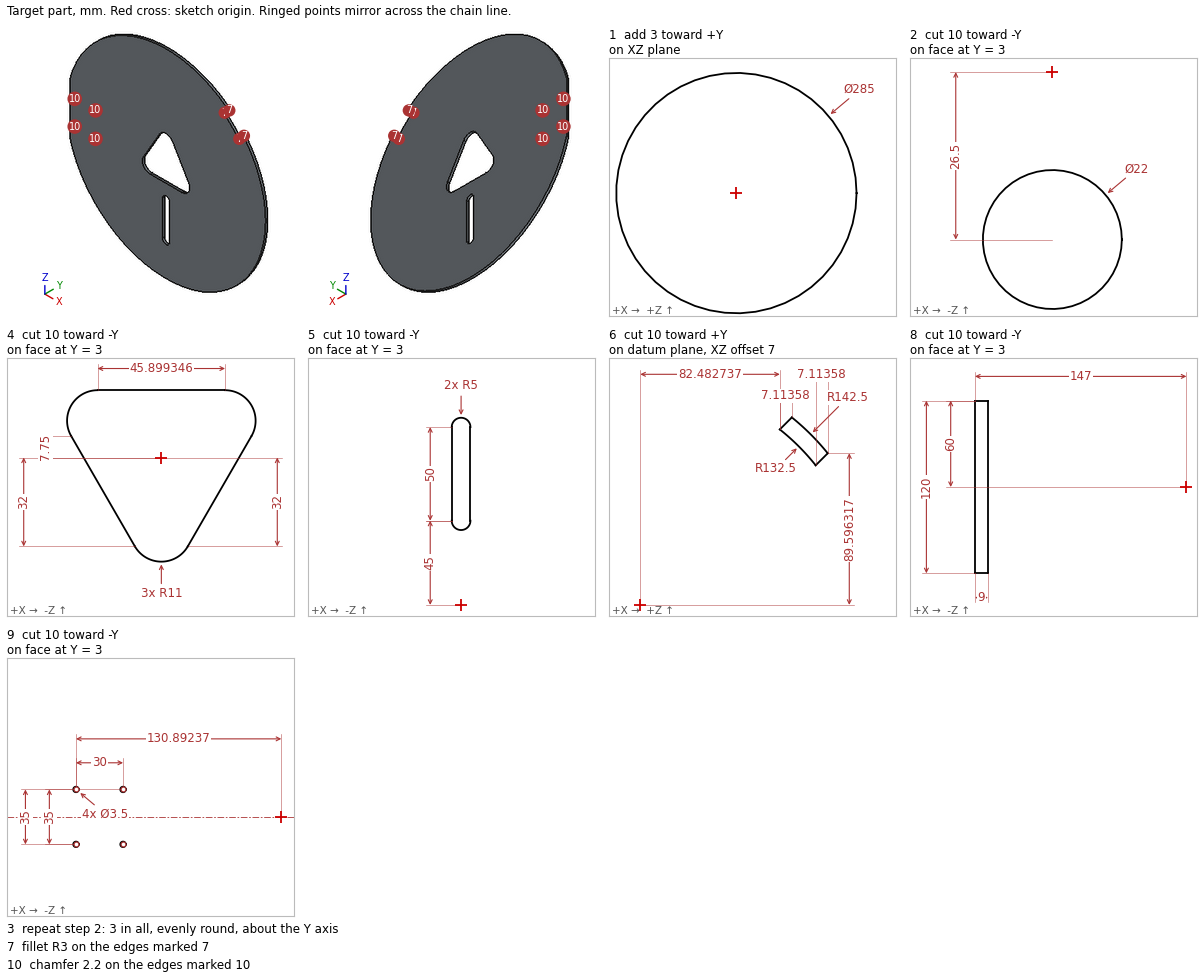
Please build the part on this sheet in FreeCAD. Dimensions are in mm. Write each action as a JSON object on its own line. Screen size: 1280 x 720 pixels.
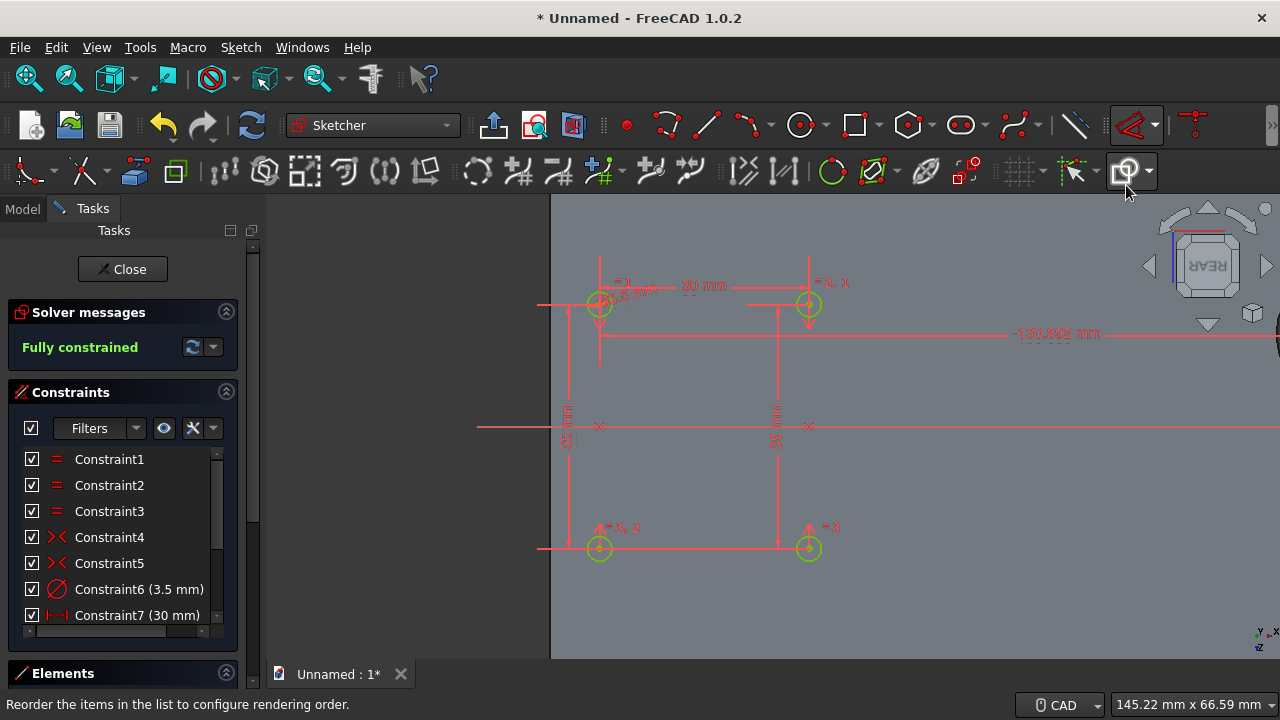
{"action": "left_click", "coordinate": [123, 269]}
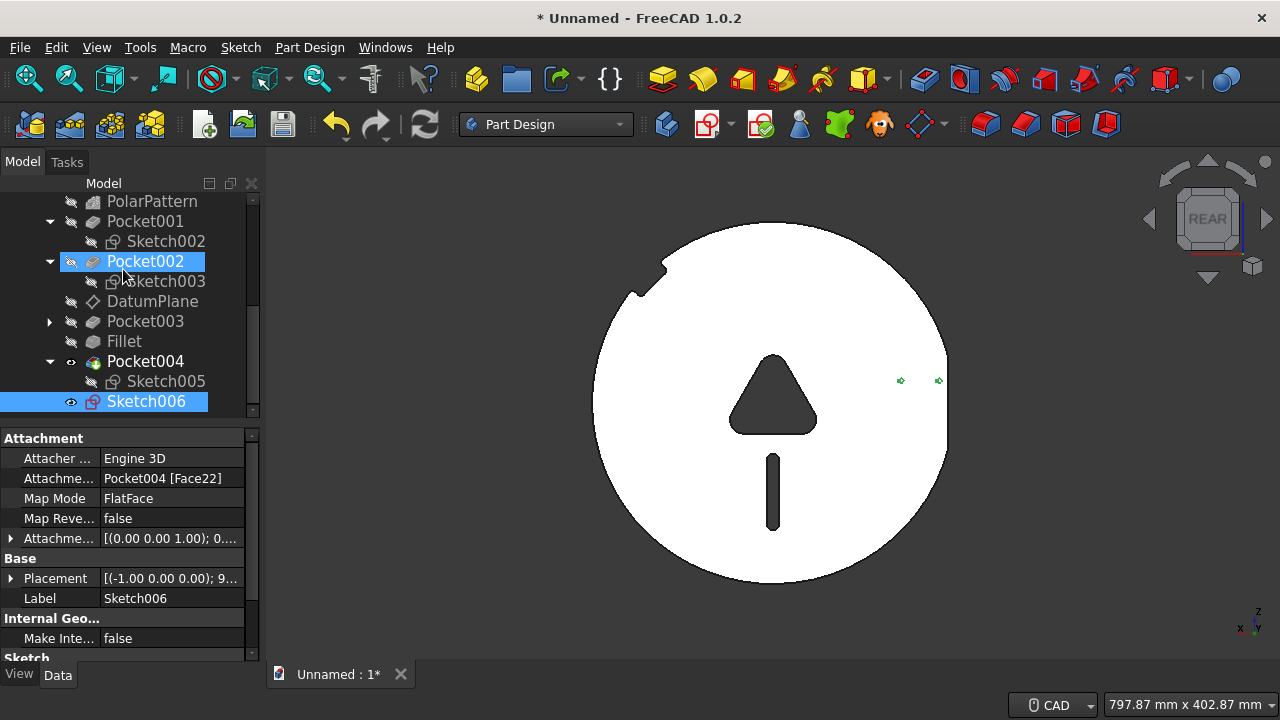
{"action": "left_click", "coordinate": [926, 80]}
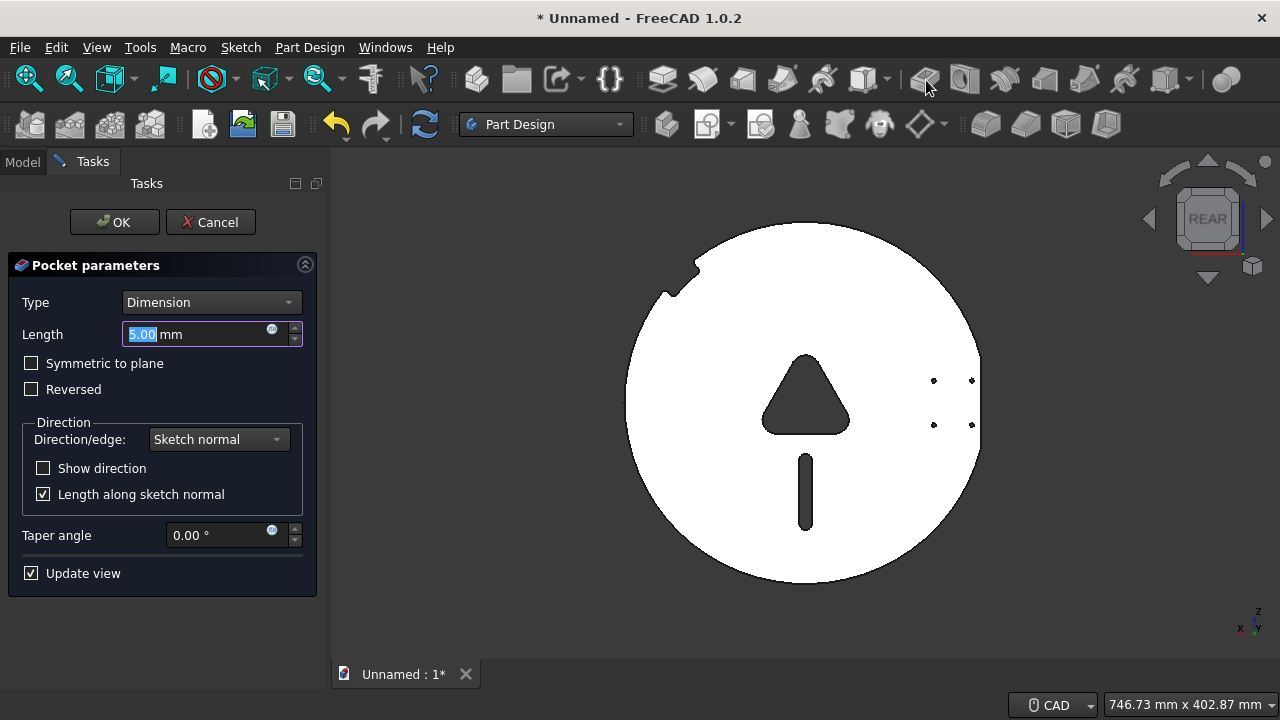
{"action": "type", "text": "10"}
{"action": "key", "text": "Tab"}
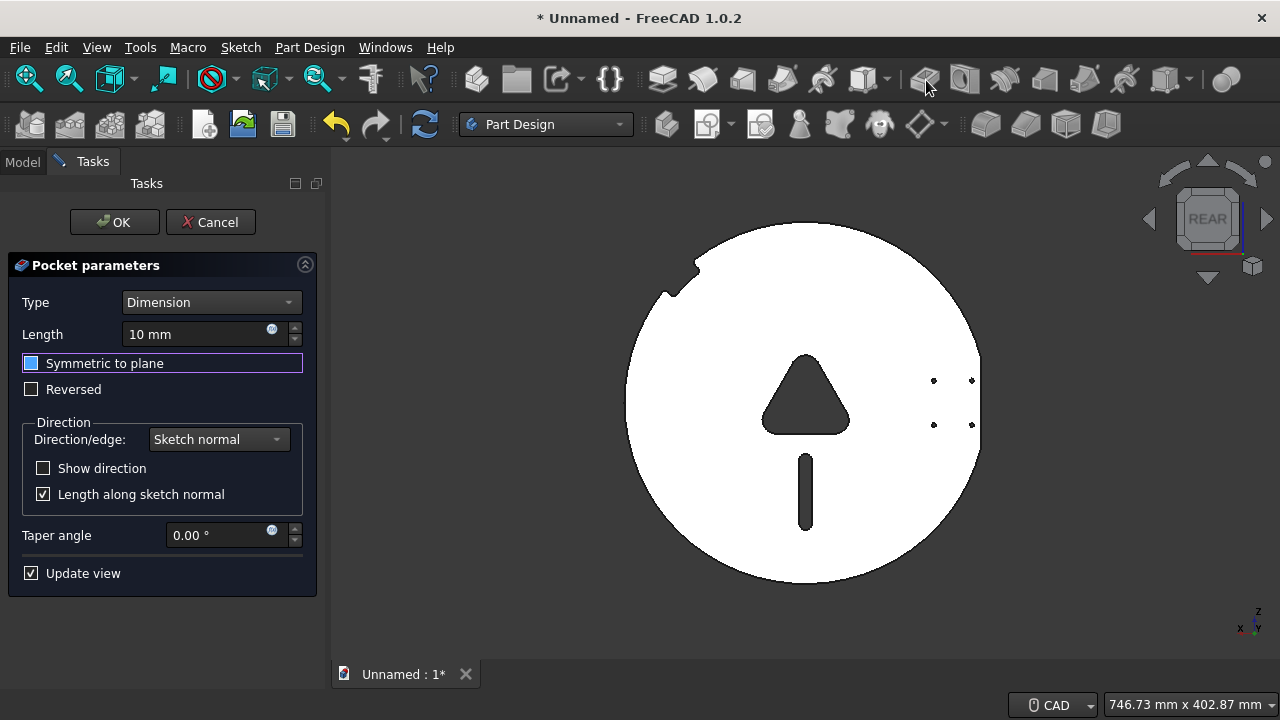
{"action": "left_click", "coordinate": [115, 222]}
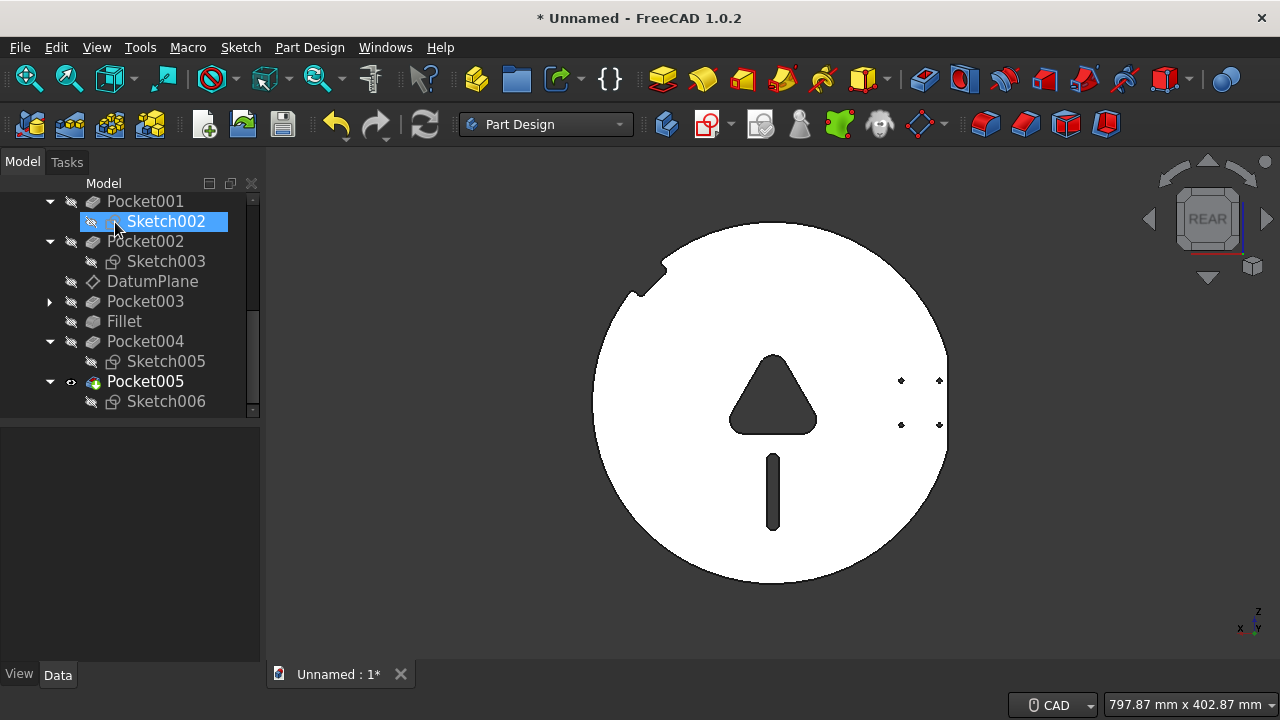
{"action": "scroll", "coordinate": [942, 424], "scroll_direction": "up", "scroll_amount": 6}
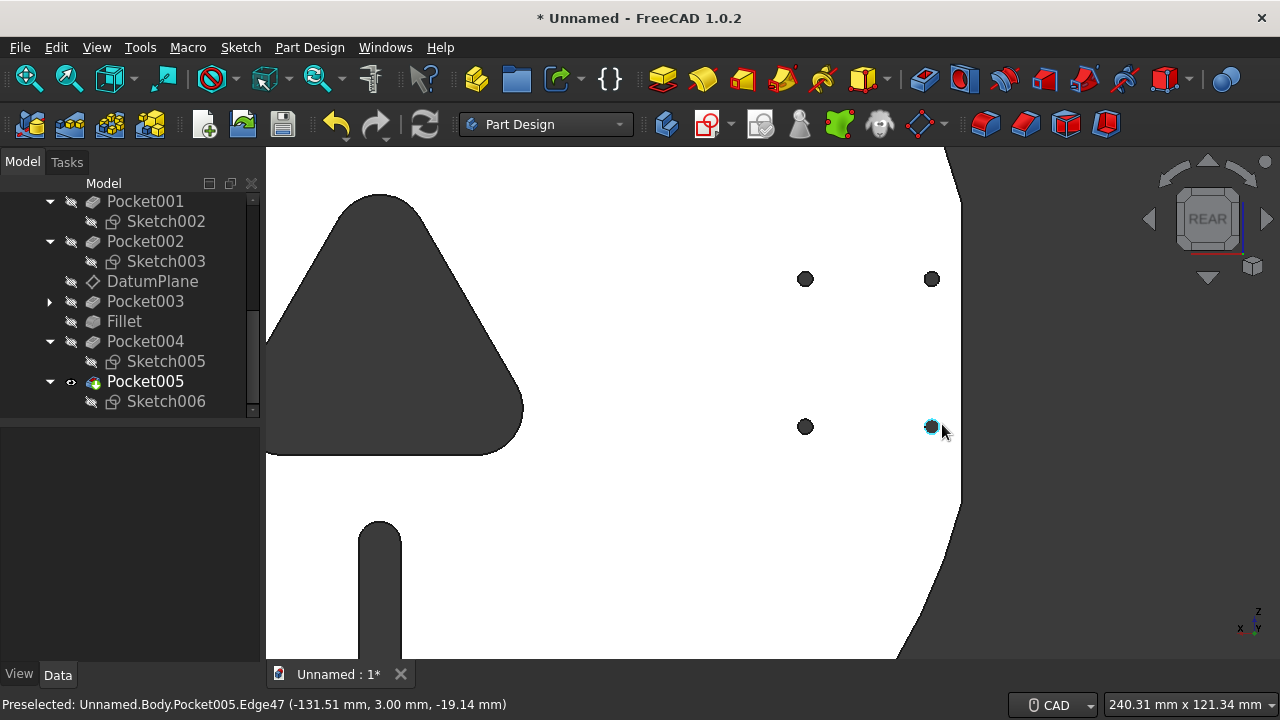
{"action": "left_click", "coordinate": [30, 80]}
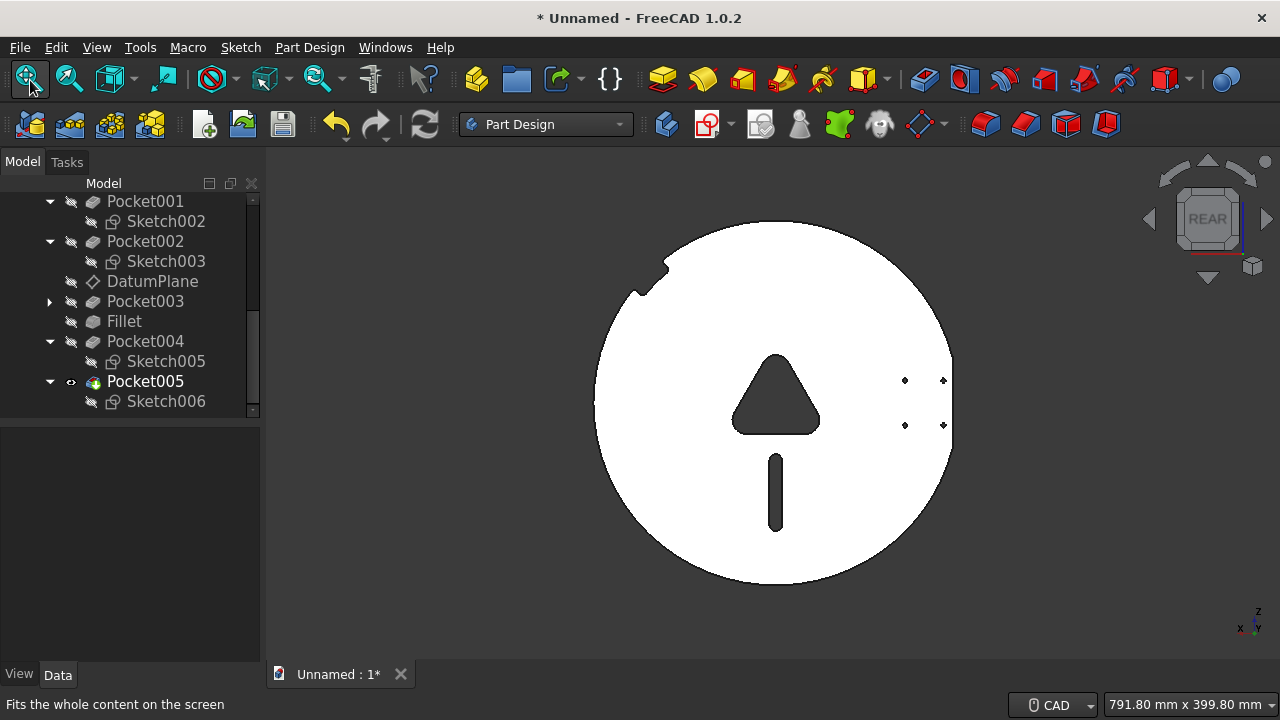
{"action": "key", "text": "0"}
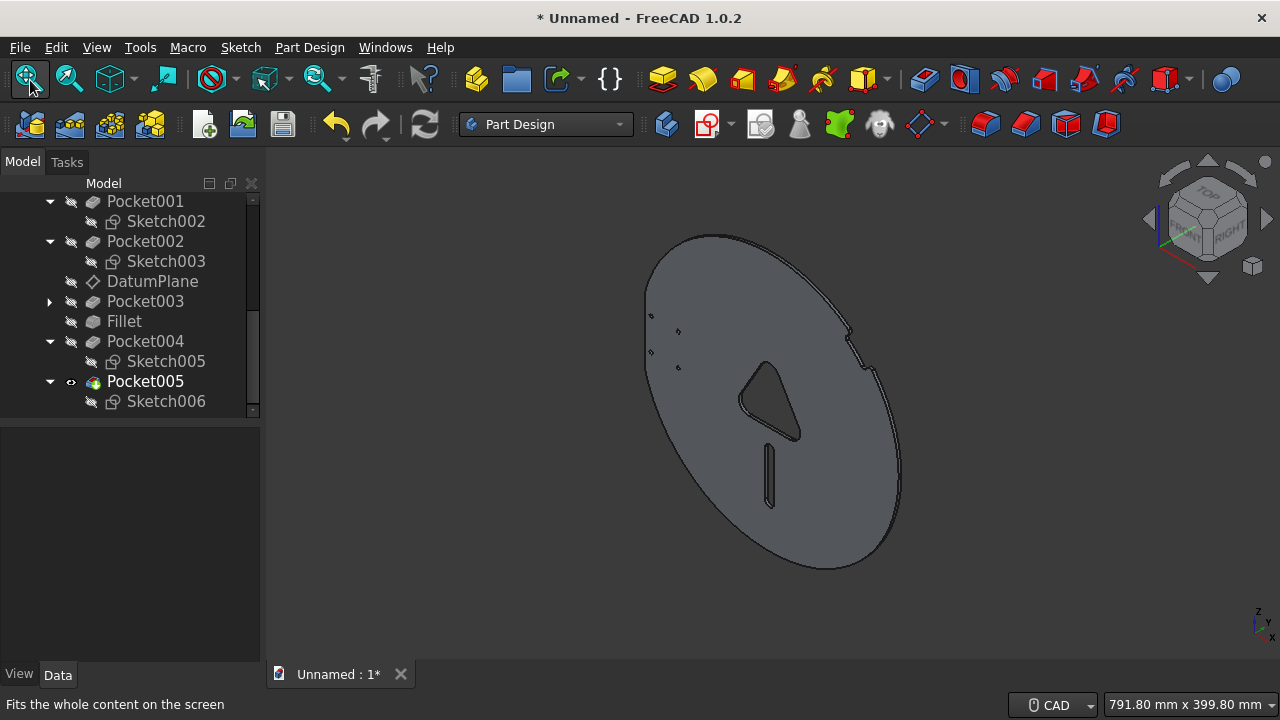
{"action": "left_click", "coordinate": [649, 351]}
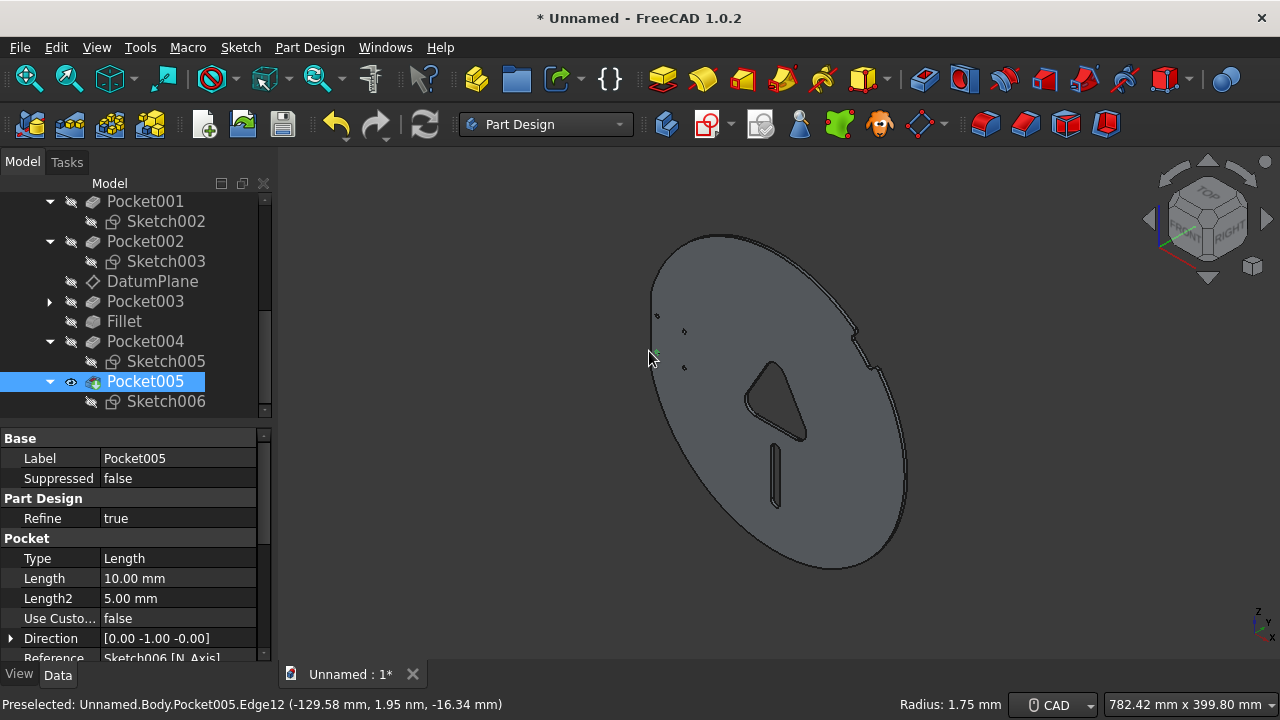
{"action": "left_click", "coordinate": [683, 366], "text": "ctrl"}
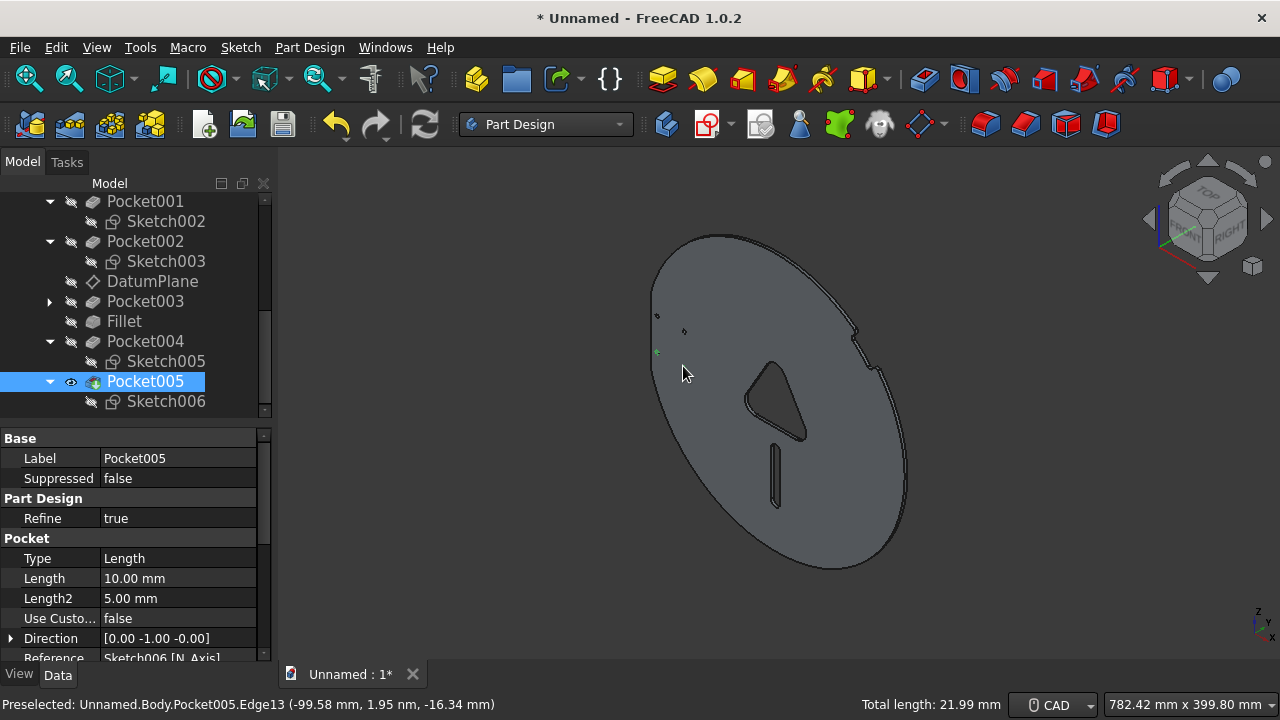
{"action": "left_click", "coordinate": [655, 314], "text": "ctrl"}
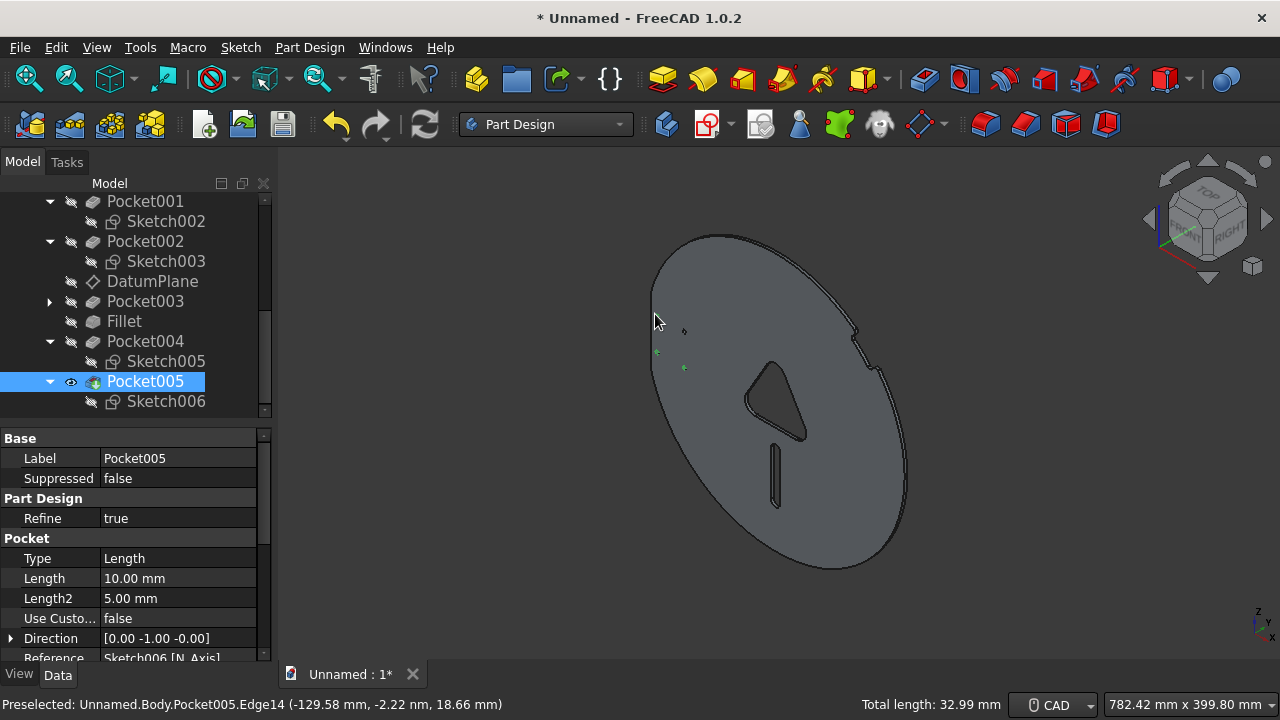
{"action": "left_click", "coordinate": [683, 330], "text": "ctrl"}